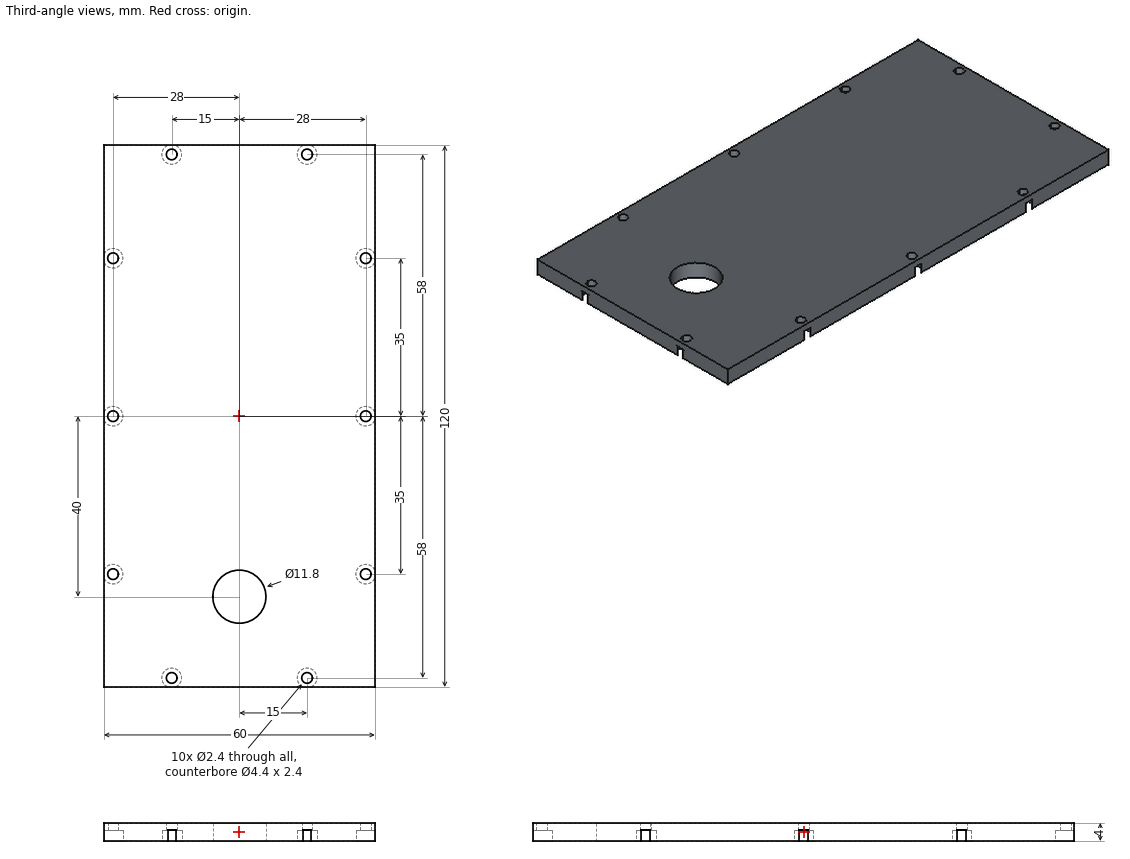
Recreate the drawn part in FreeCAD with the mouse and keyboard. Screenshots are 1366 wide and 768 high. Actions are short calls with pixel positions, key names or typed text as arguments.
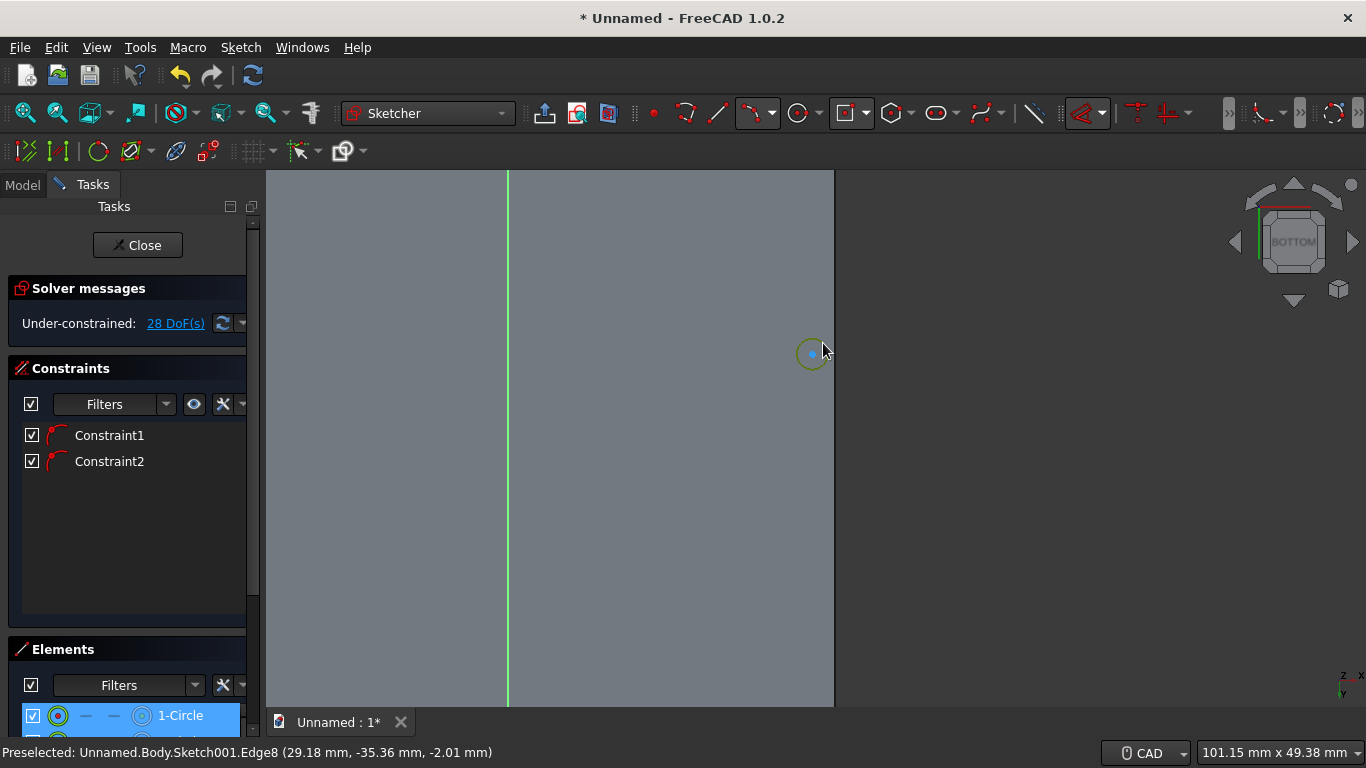
scroll(826, 343, down, 7)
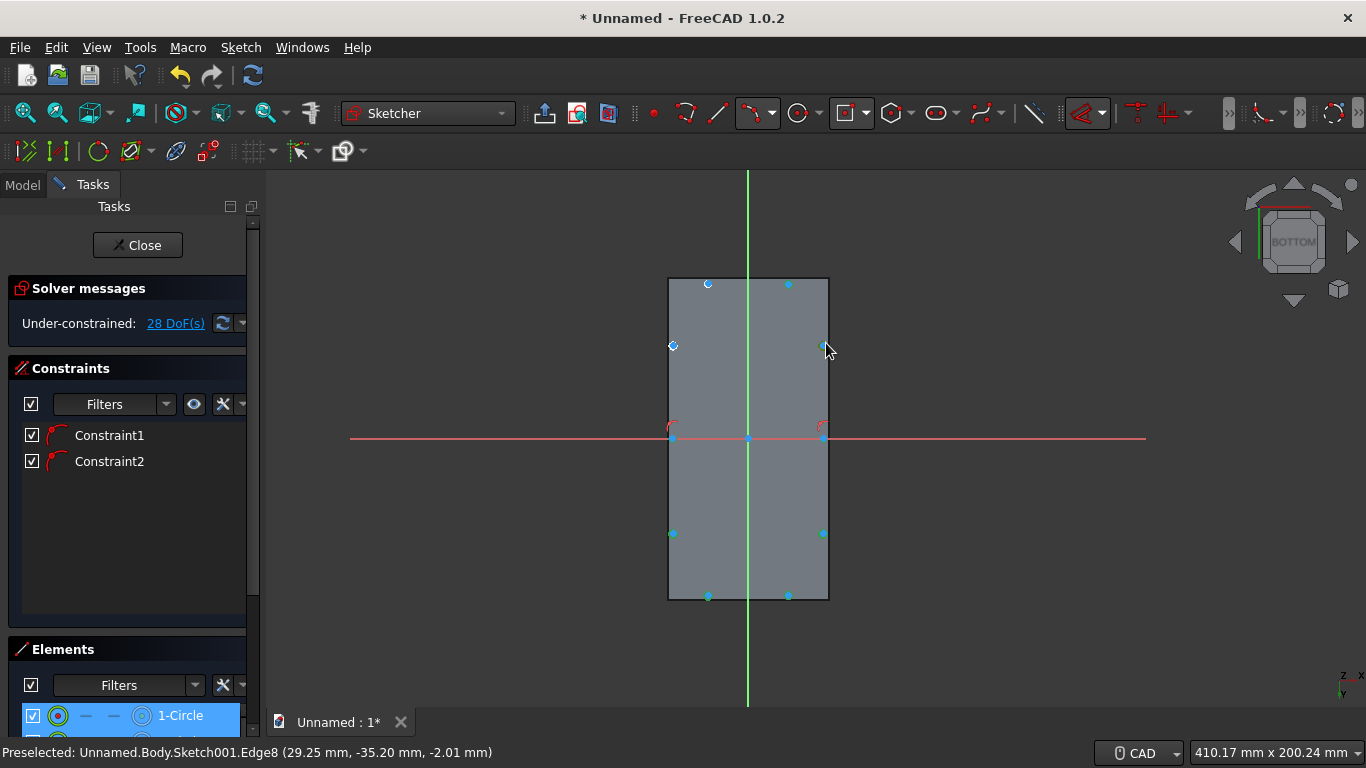
scroll(676, 343, up, 7)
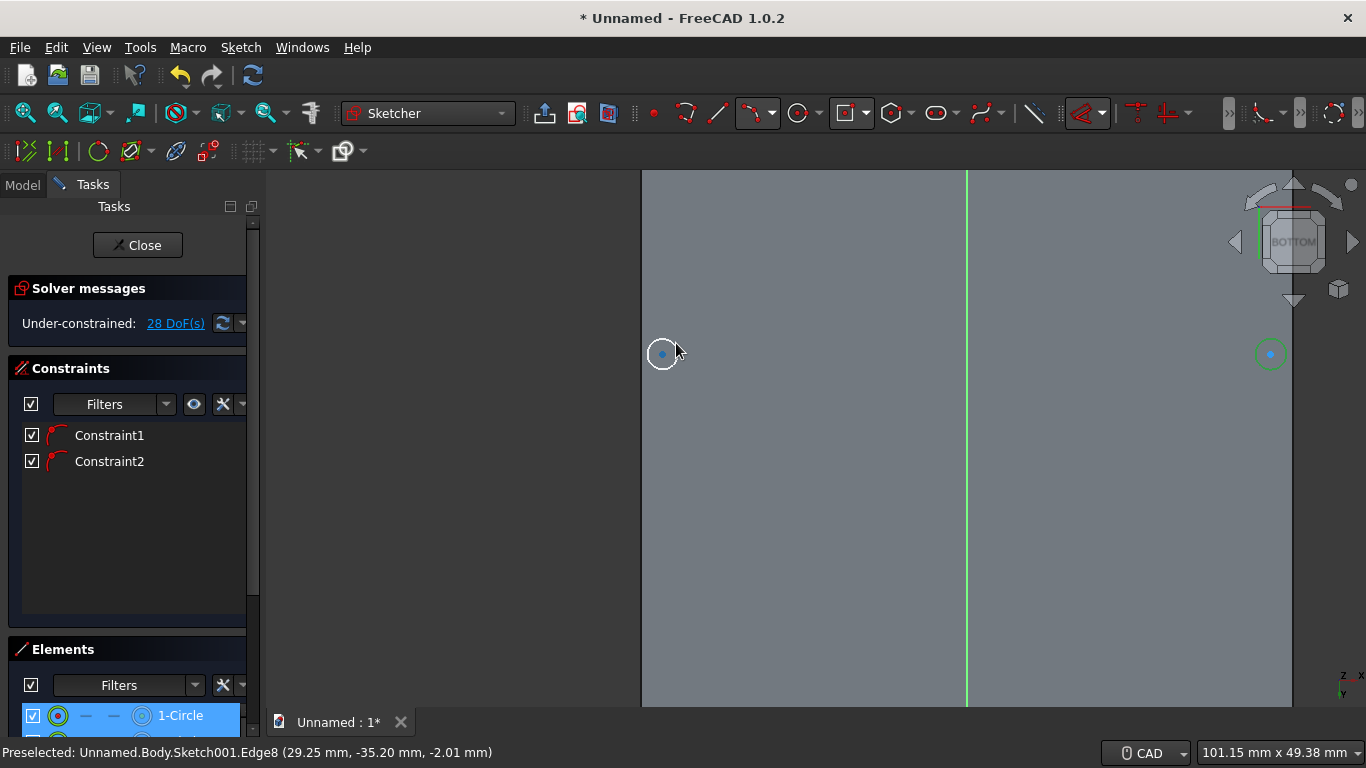
click(673, 343)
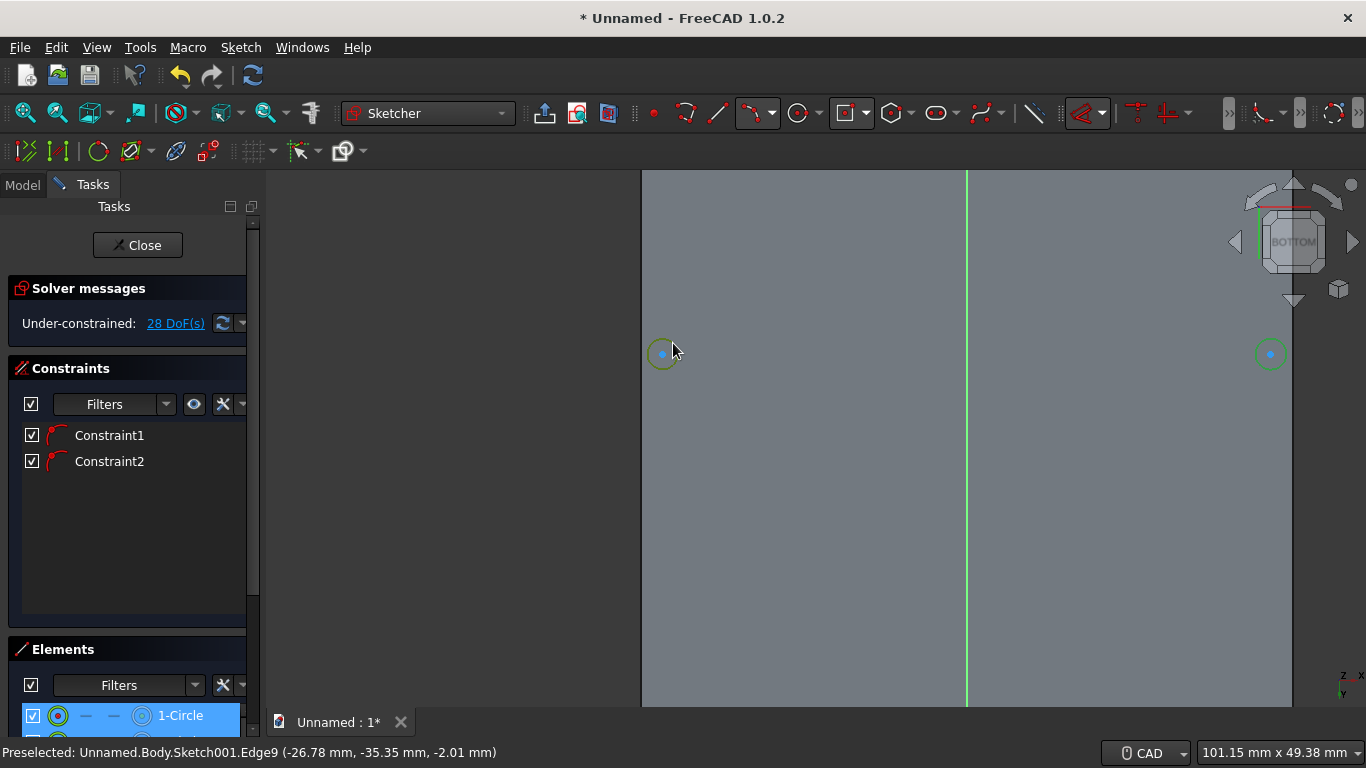
scroll(676, 343, down, 7)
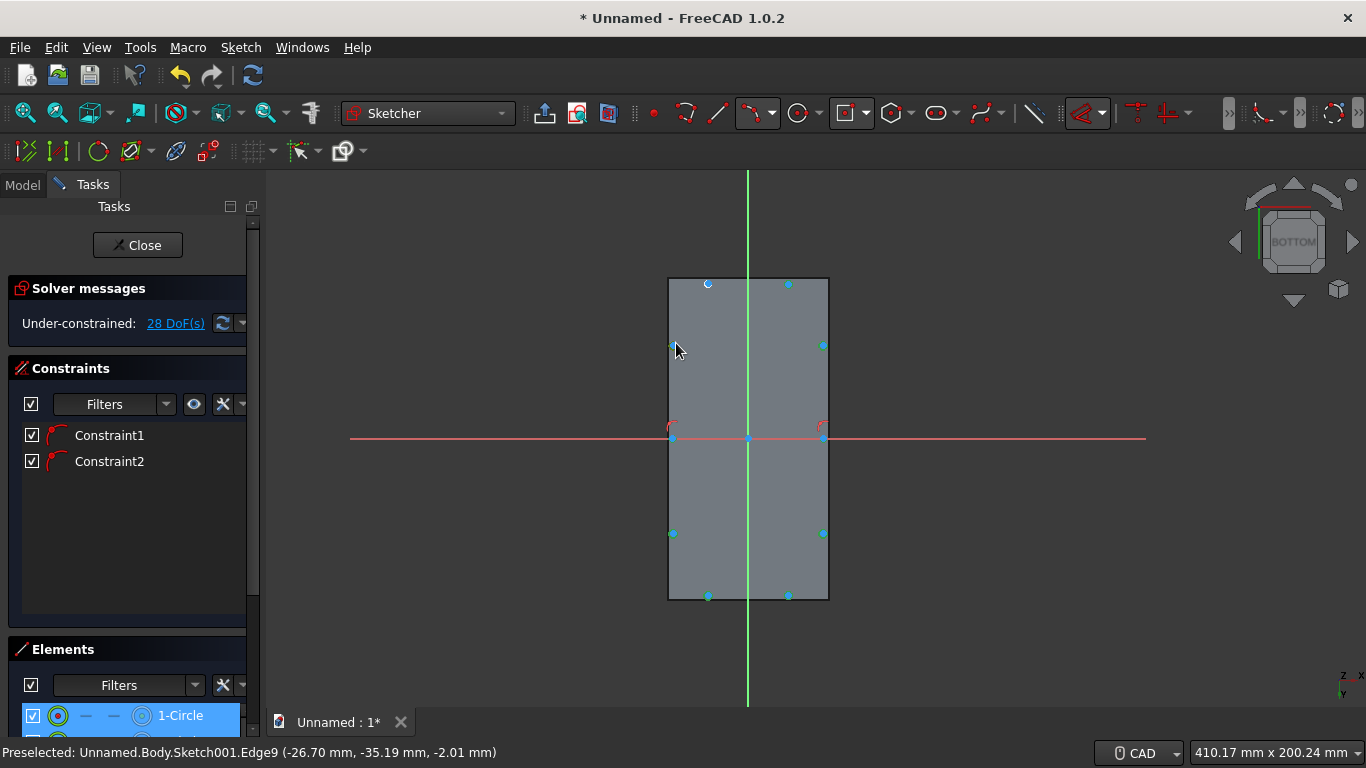
scroll(710, 282, up, 8)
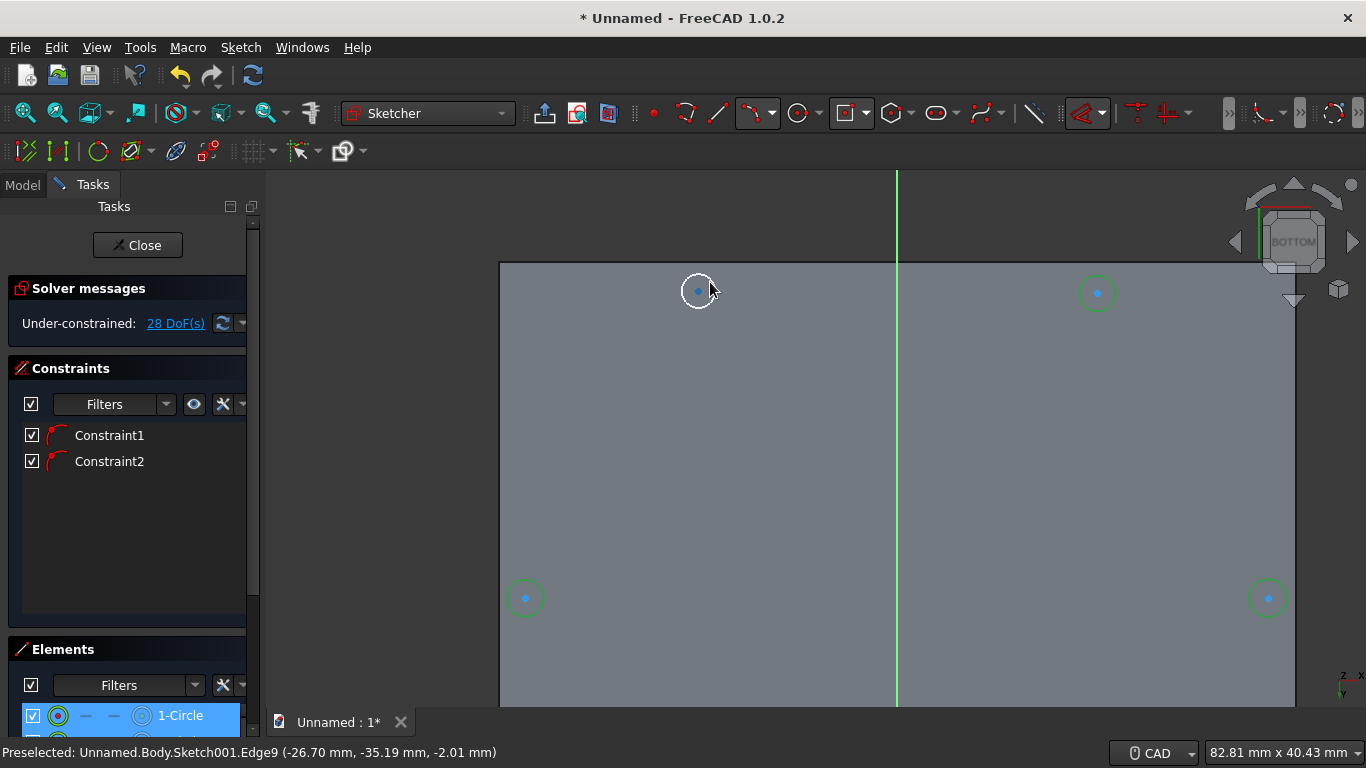
click(710, 279)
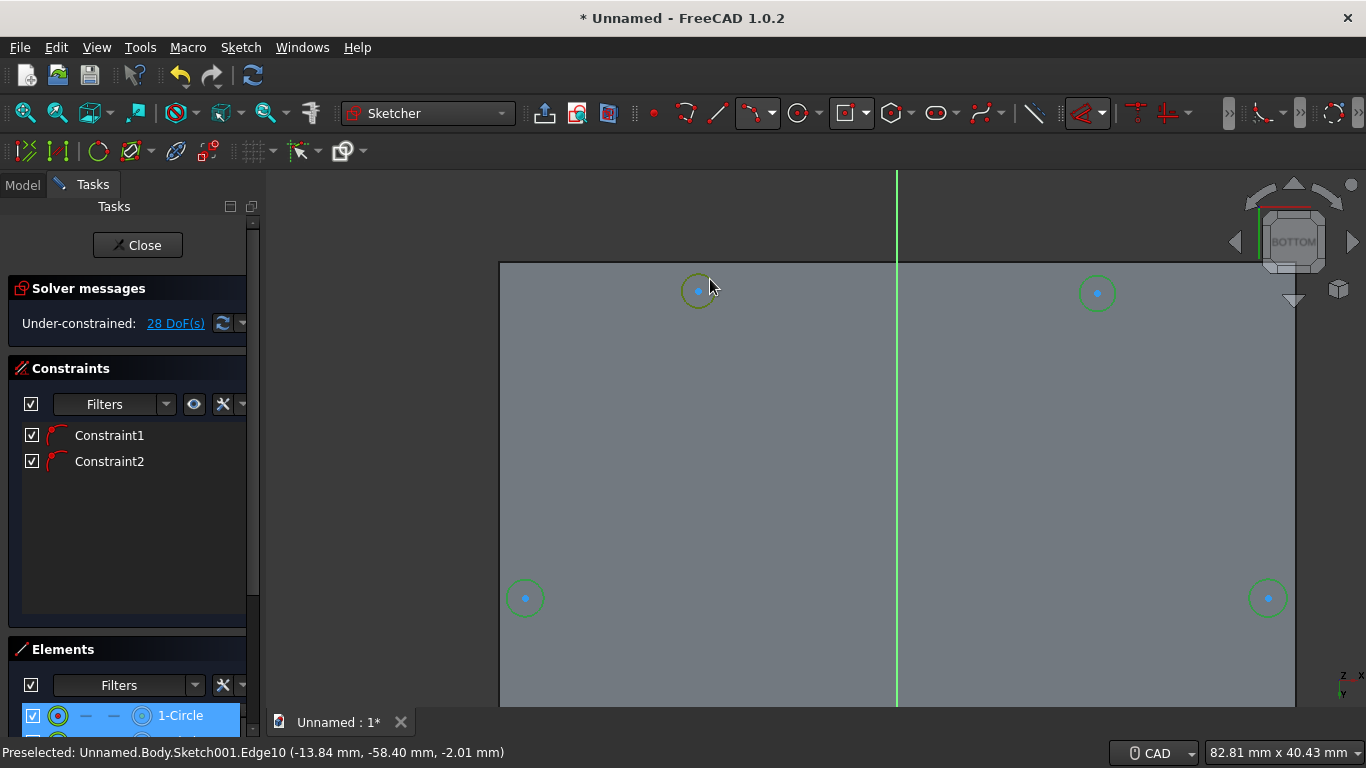
key(e)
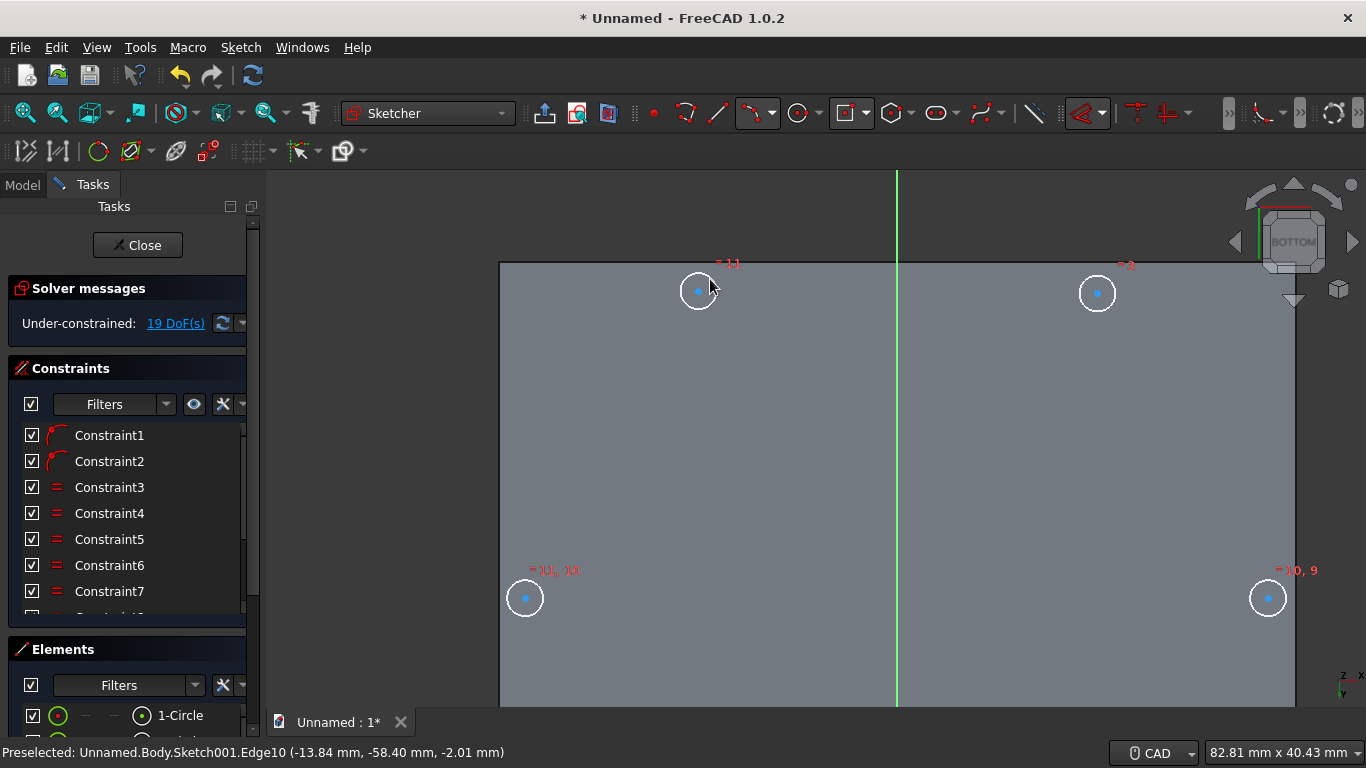
scroll(710, 282, down, 8)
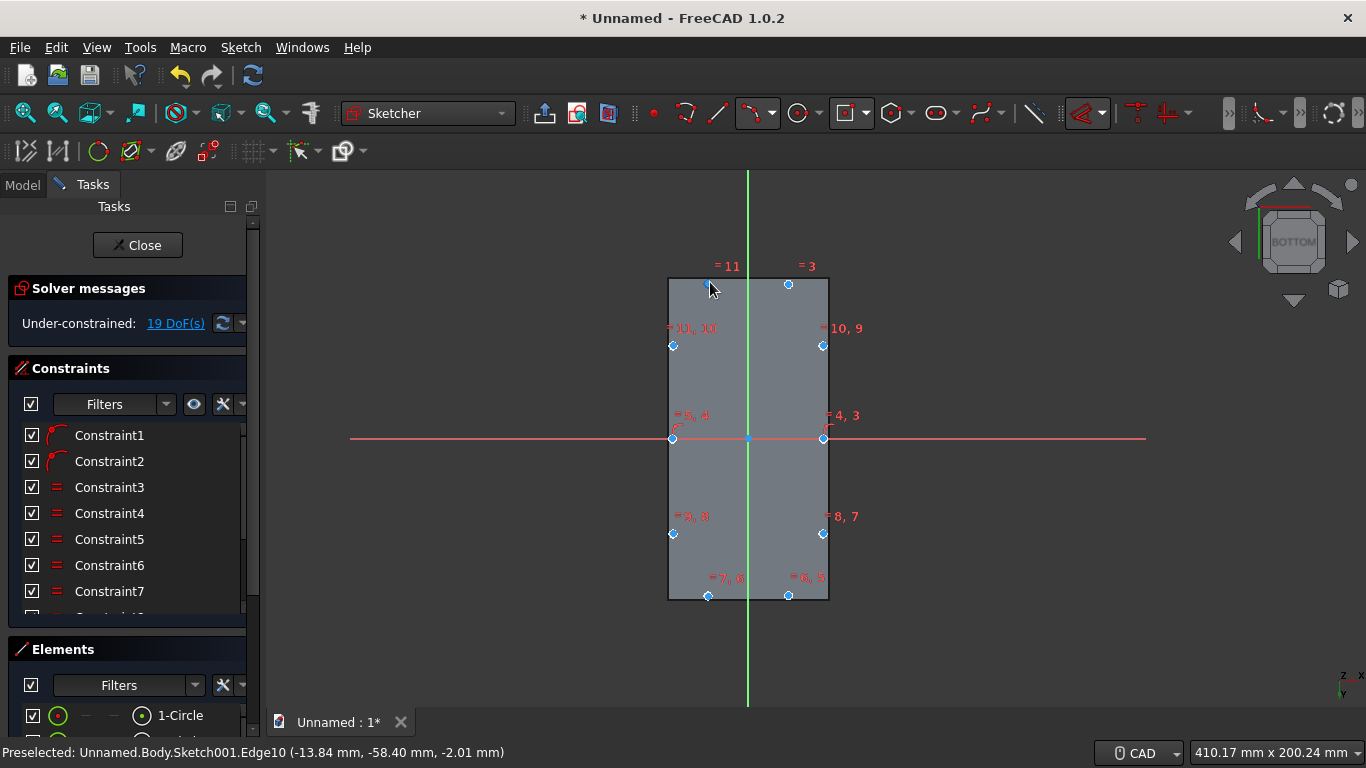
click(789, 284)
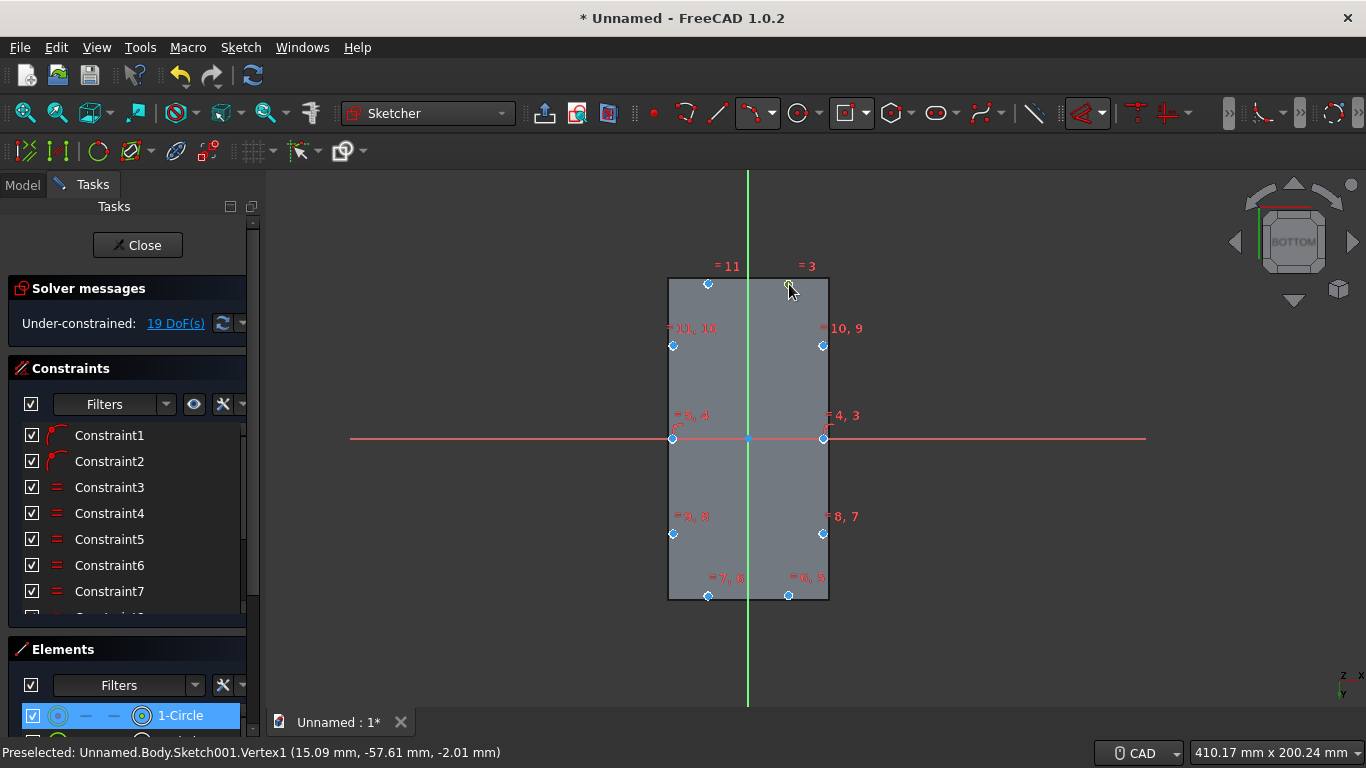
click(789, 596)